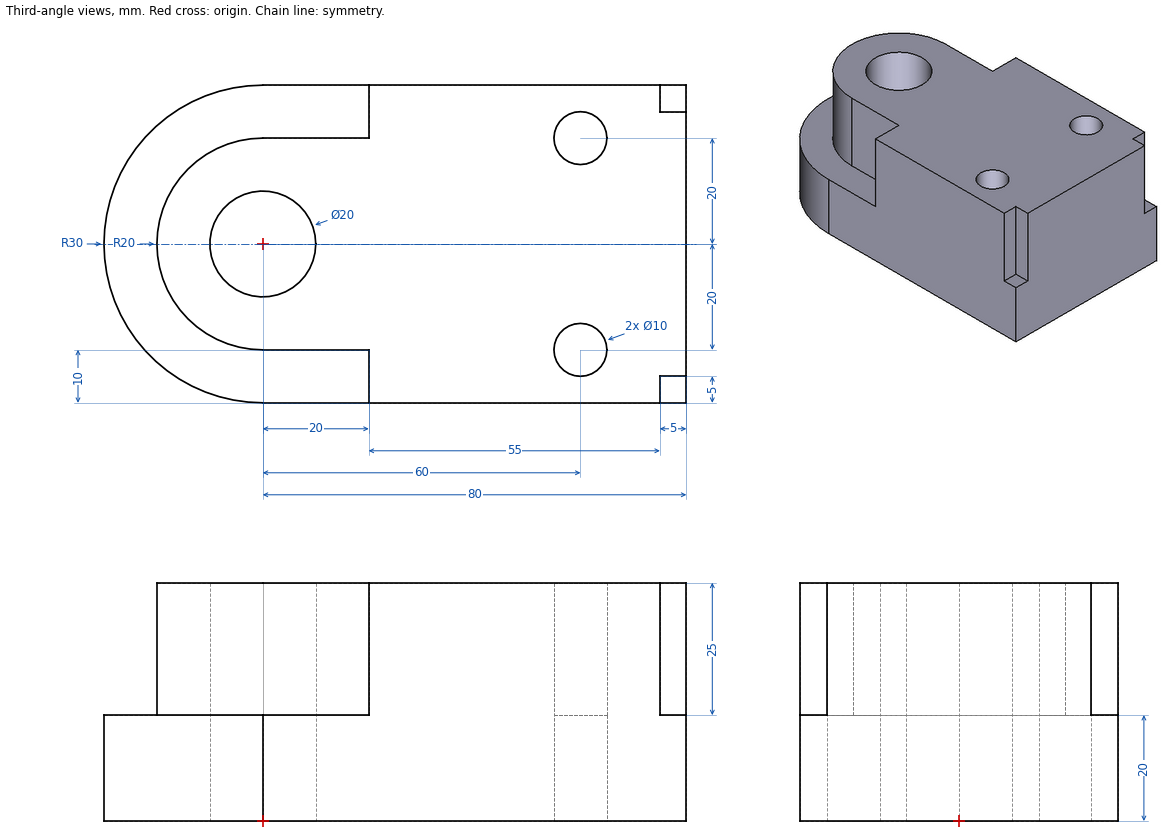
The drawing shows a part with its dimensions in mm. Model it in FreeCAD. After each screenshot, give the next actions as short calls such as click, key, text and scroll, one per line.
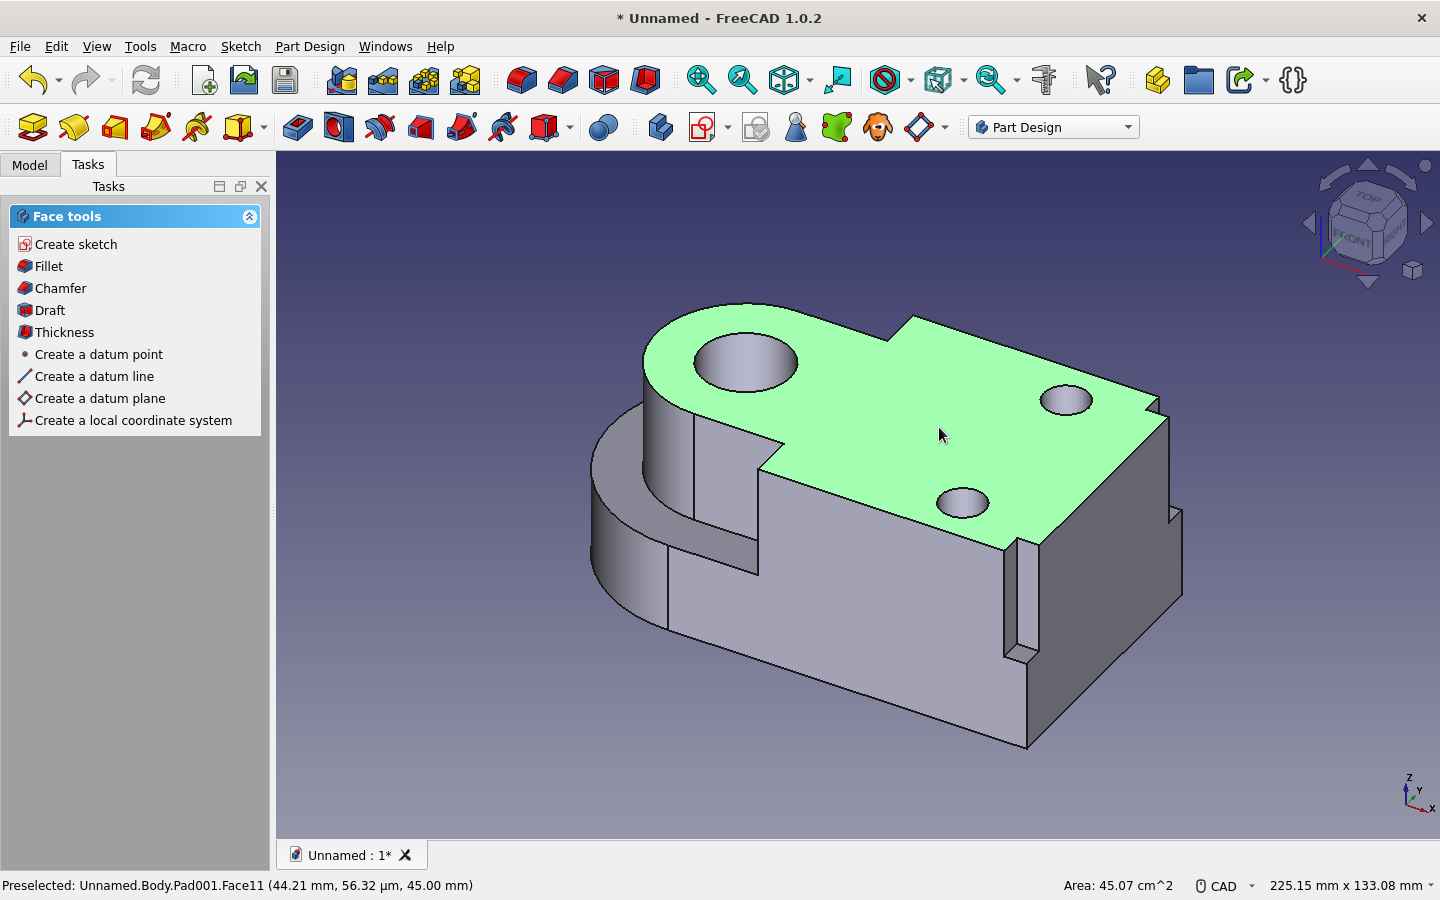
click(702, 128)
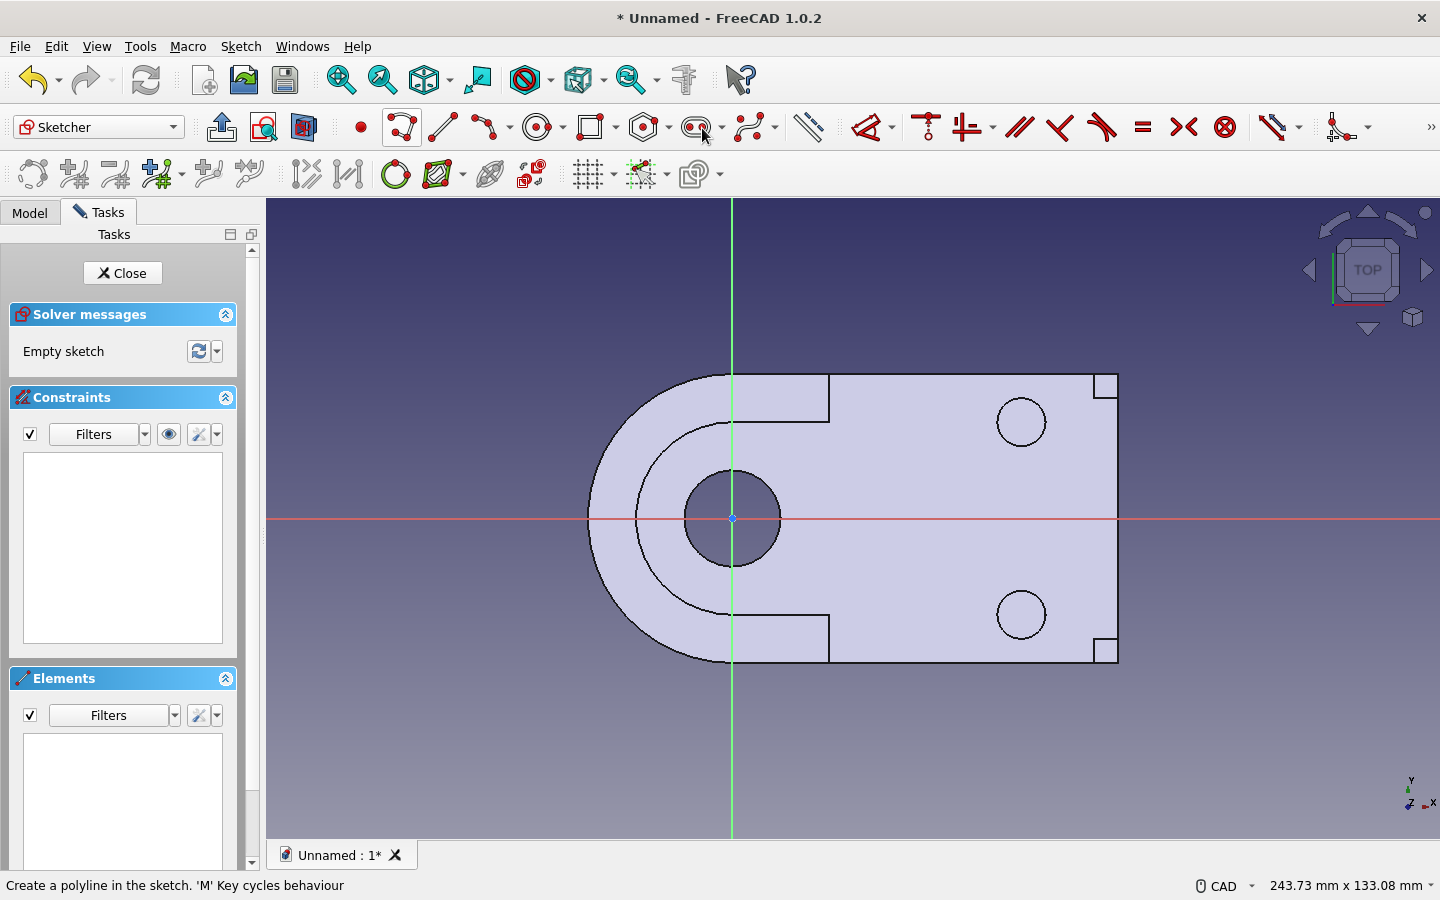
scroll(1016, 518, up, 3)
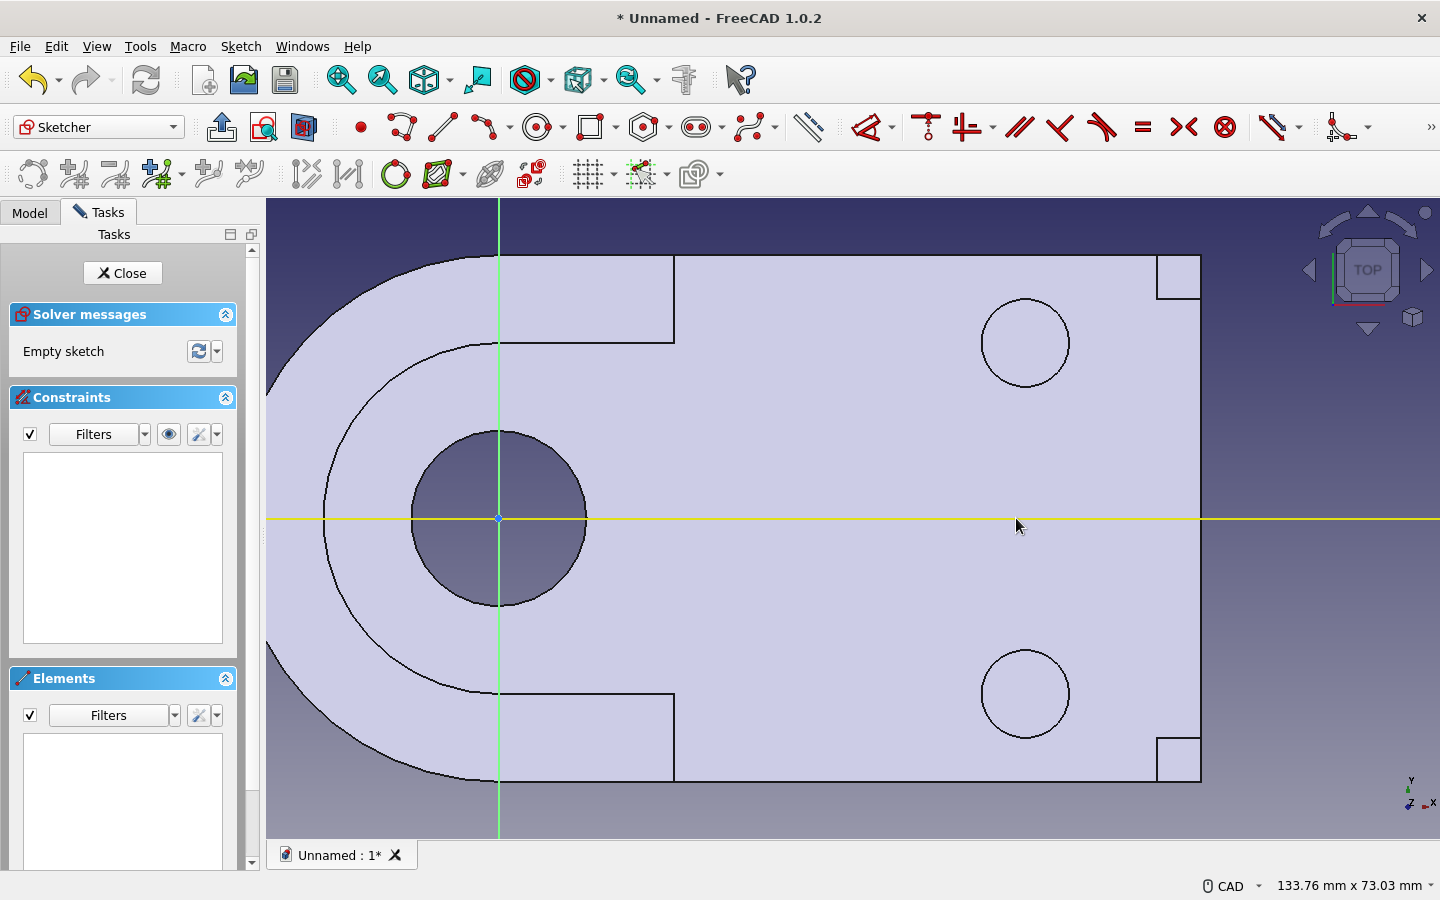
click(536, 128)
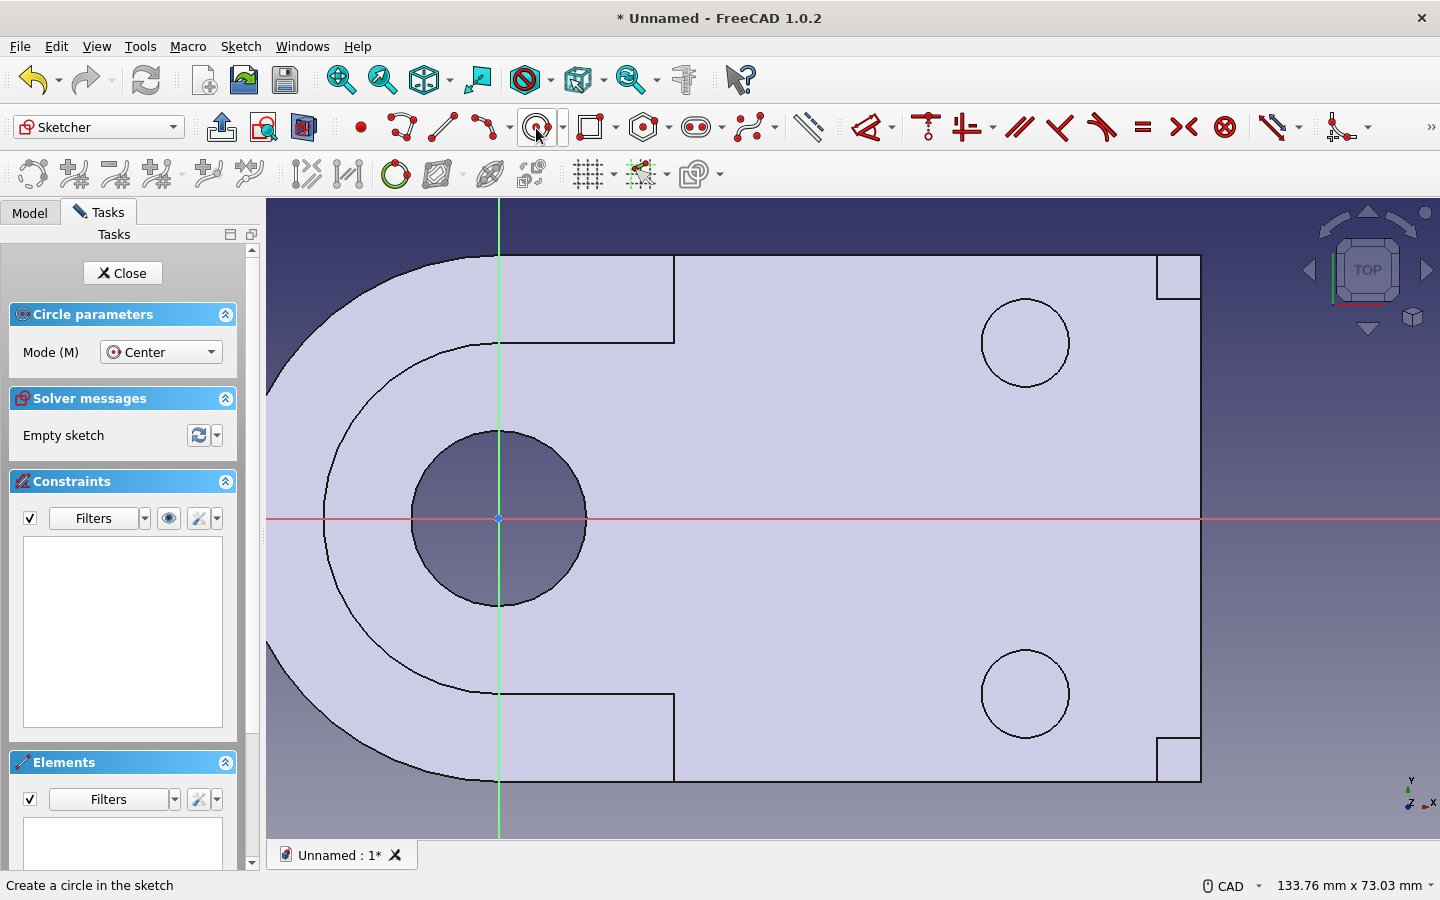
click(1025, 694)
move(1056, 663)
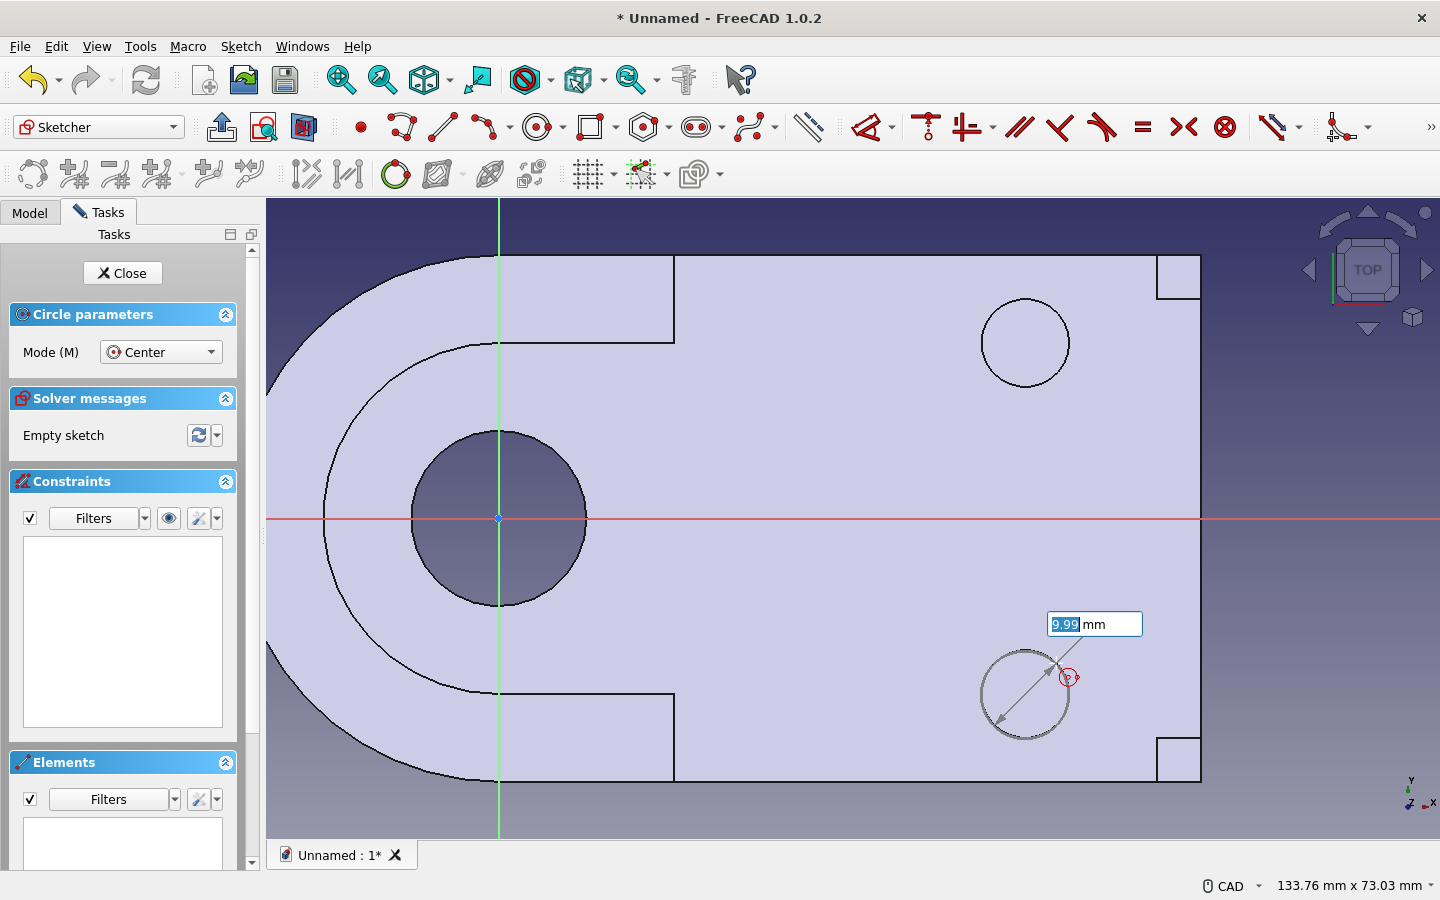
text(10)
key(Return)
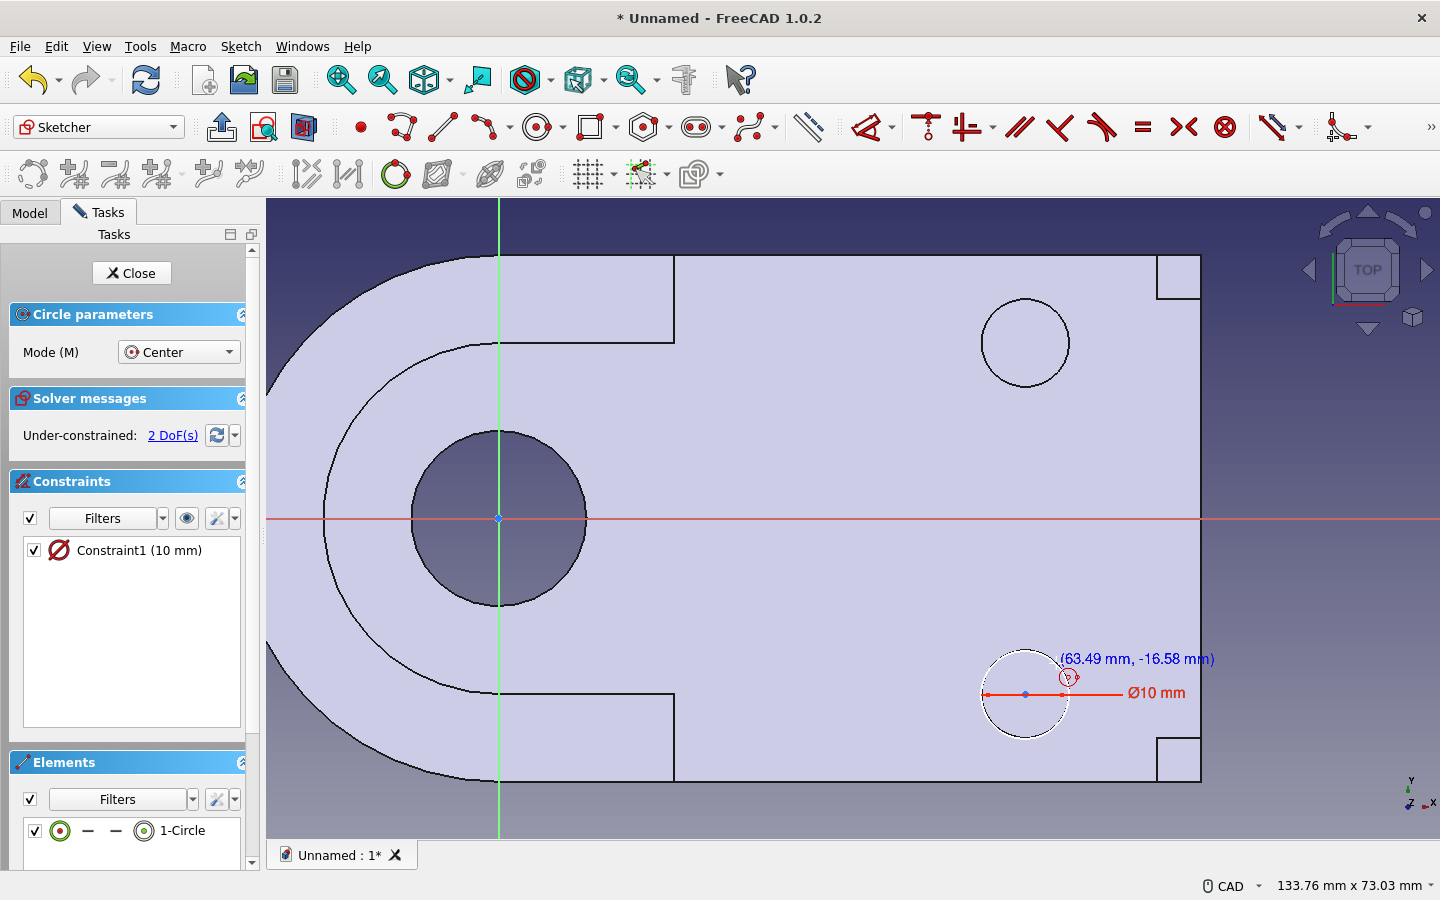
click(1025, 343)
move(1056, 312)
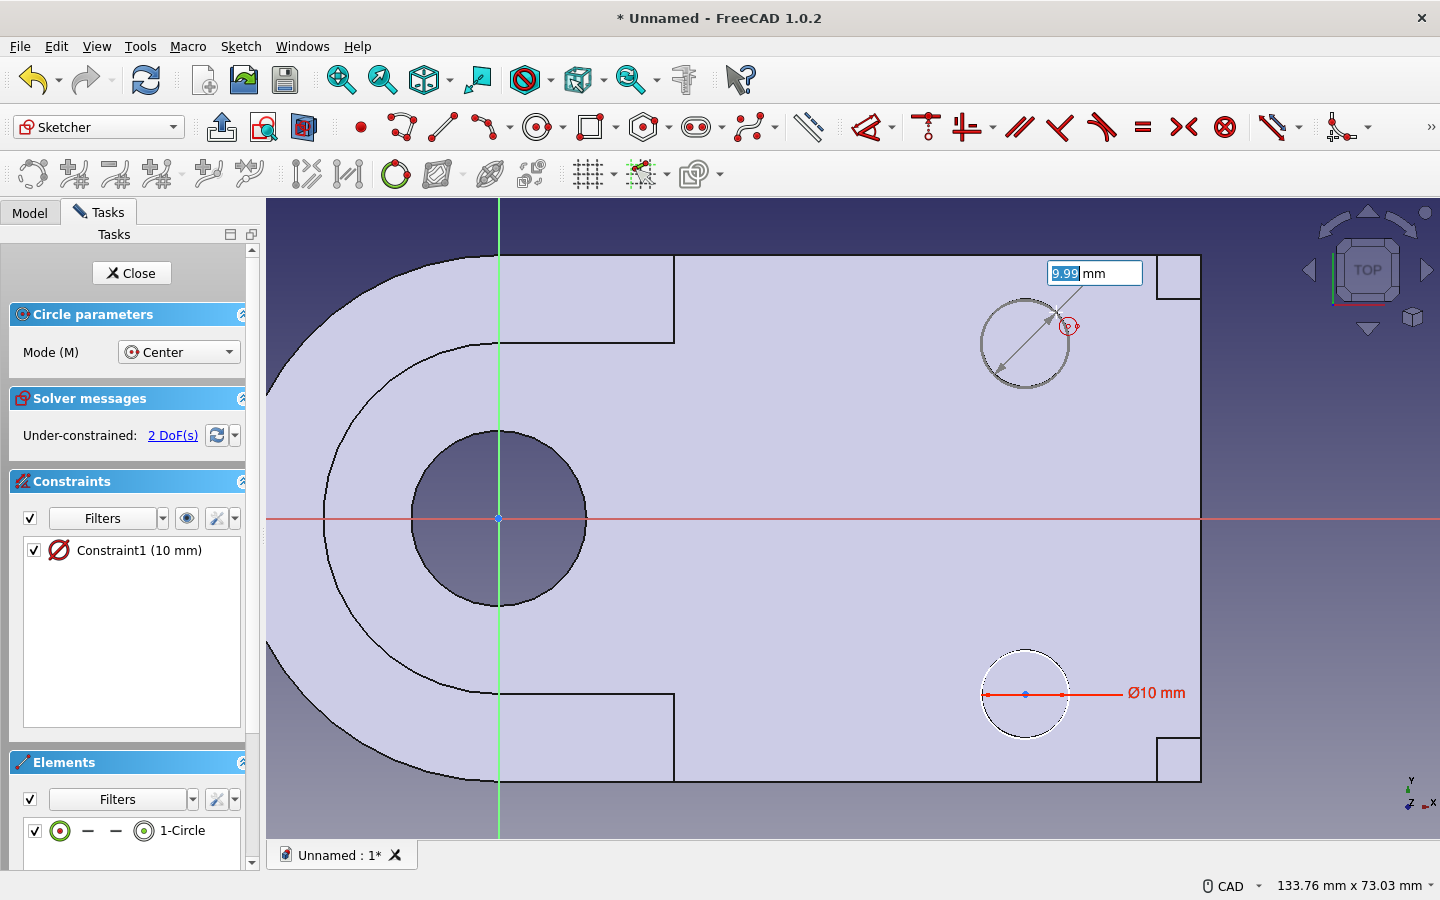
text(10)
key(Return)
key(Escape)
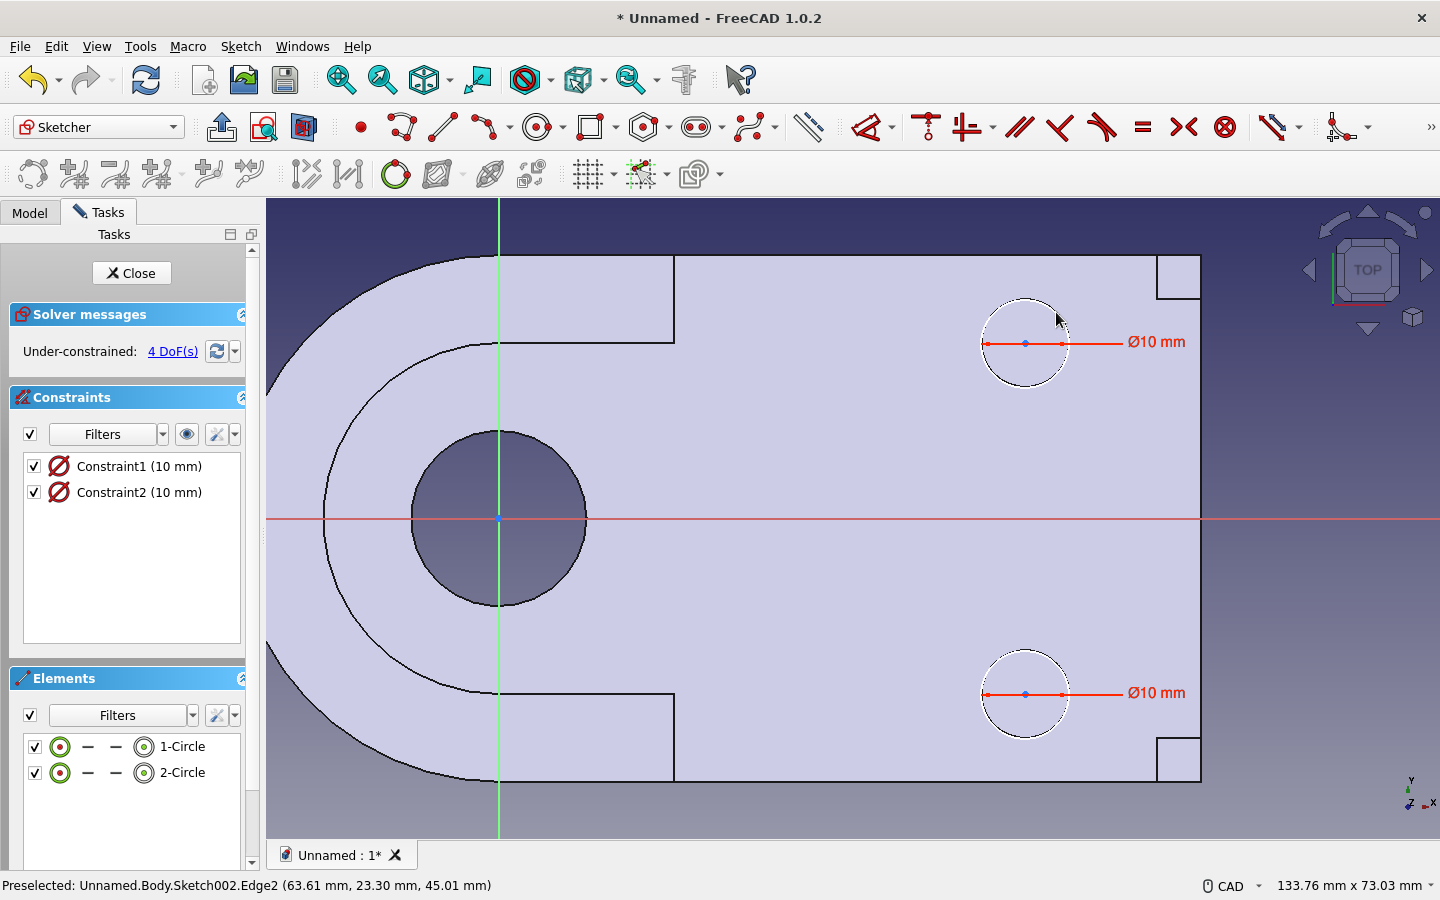
click(1025, 695)